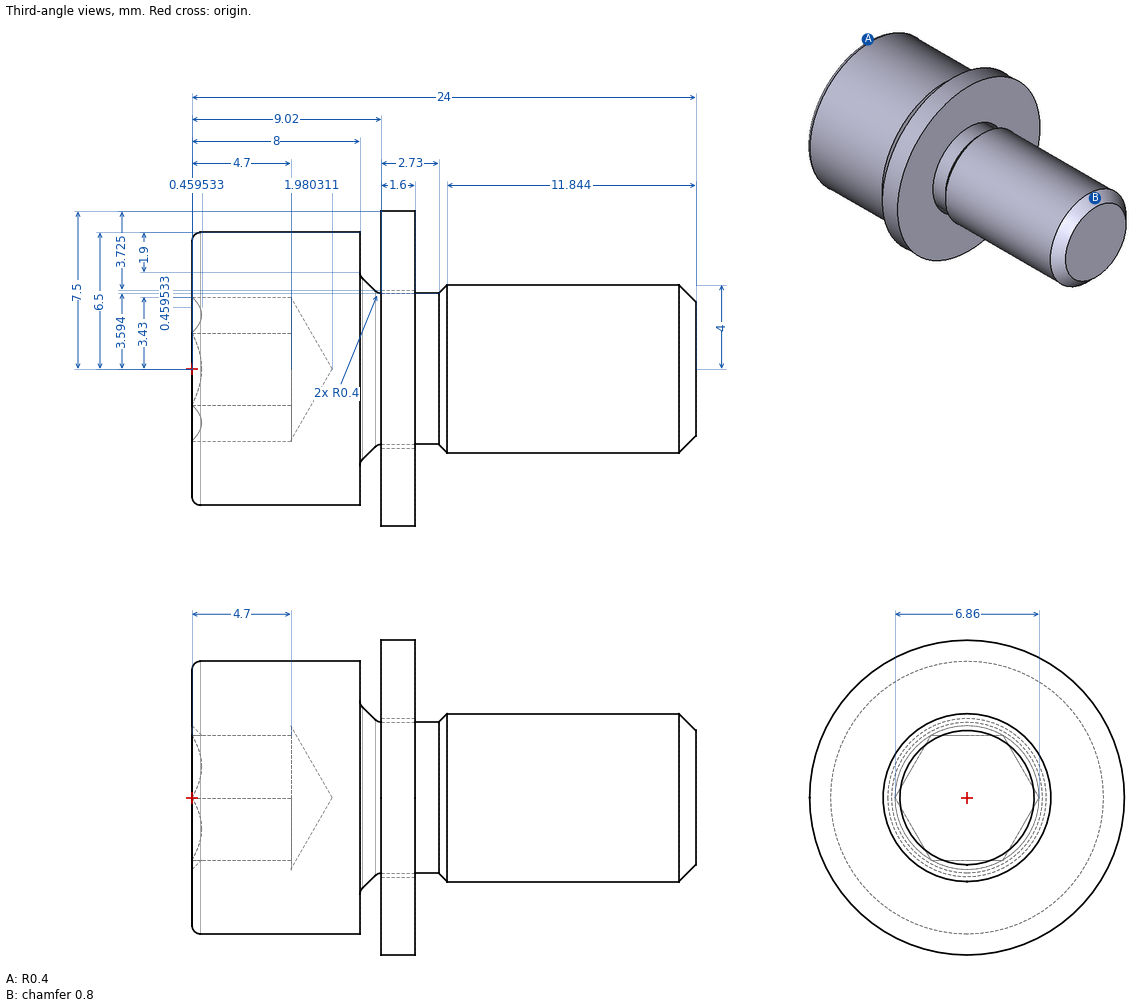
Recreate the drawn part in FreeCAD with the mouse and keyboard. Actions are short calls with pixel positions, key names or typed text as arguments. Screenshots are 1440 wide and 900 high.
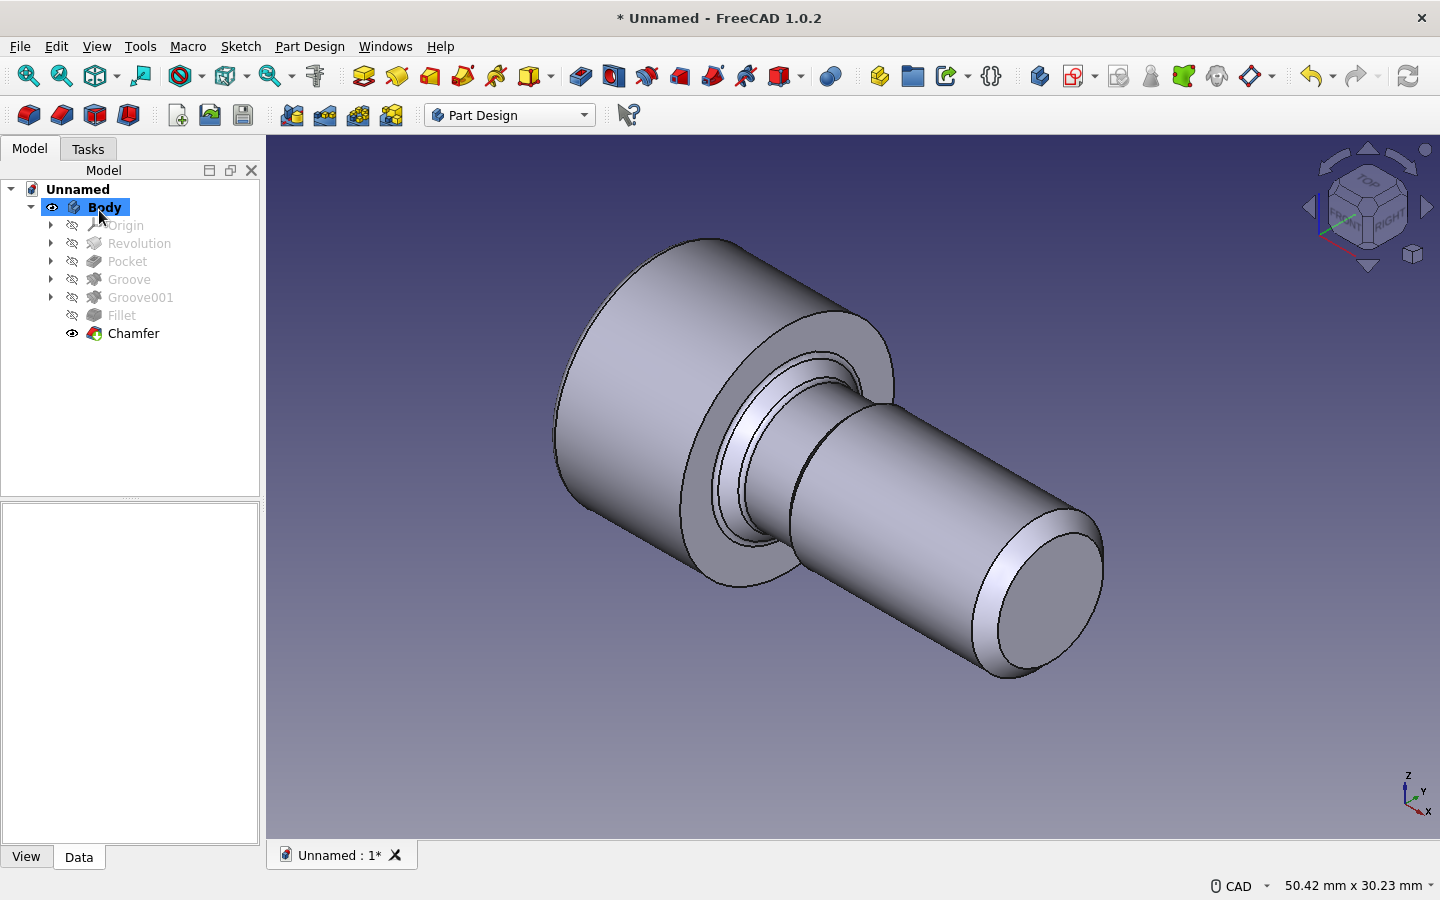
click(1040, 76)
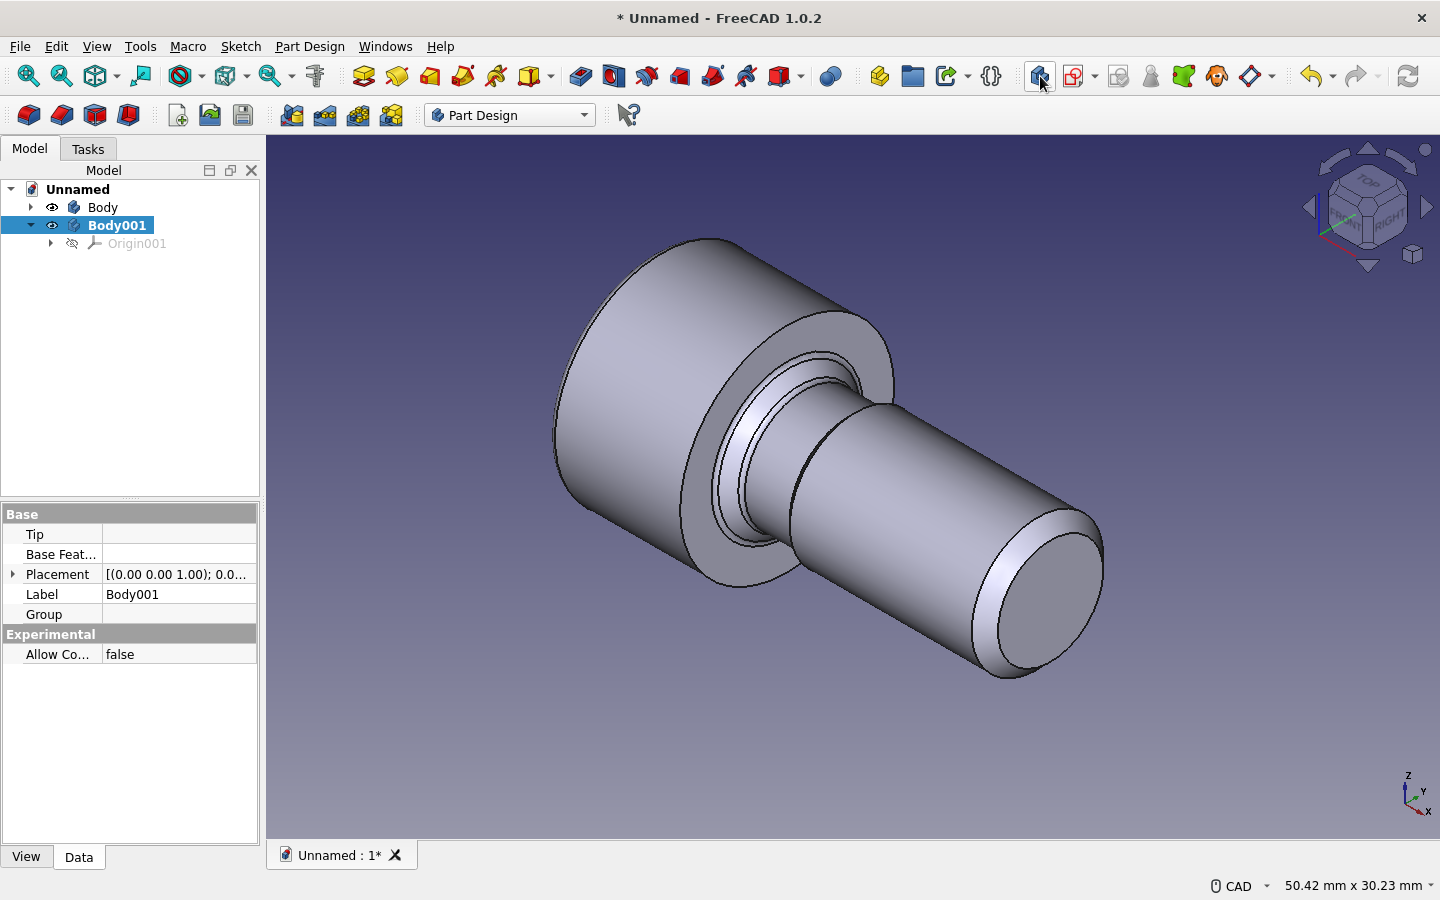
click(306, 799)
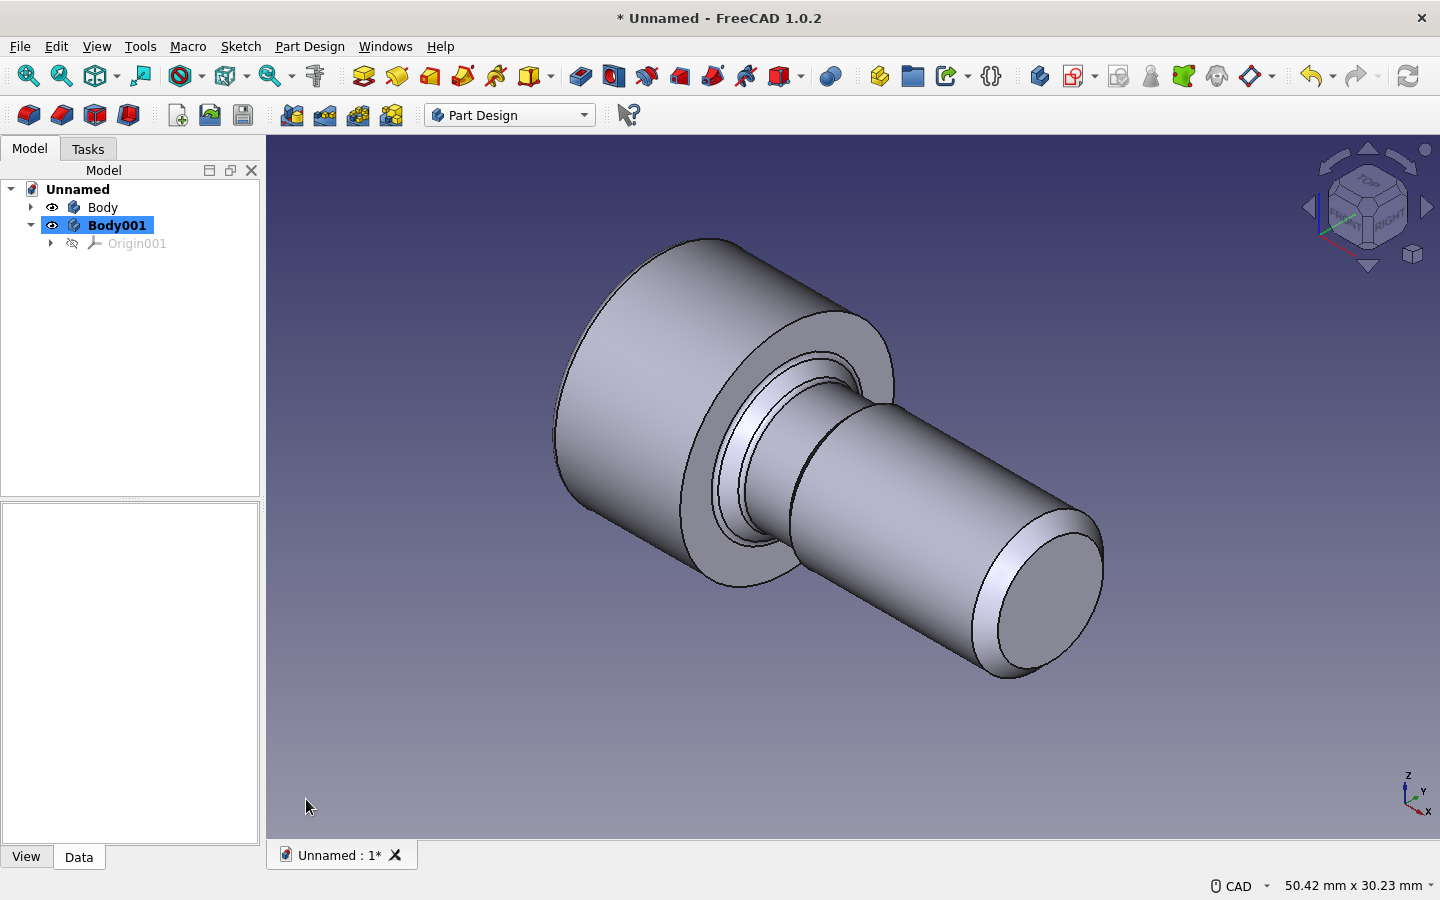
click(1072, 76)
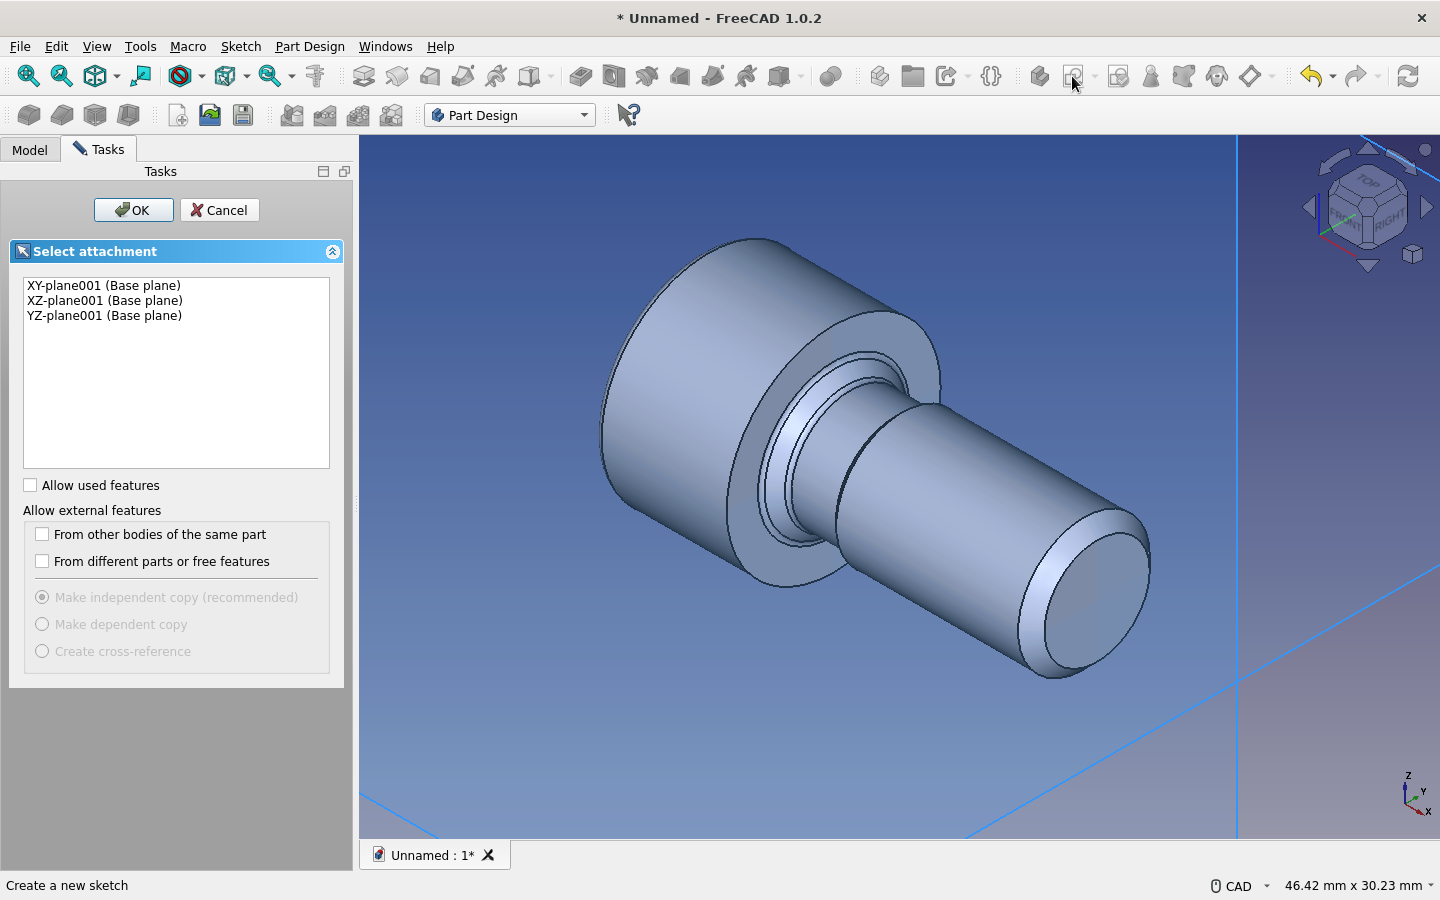
click(84, 286)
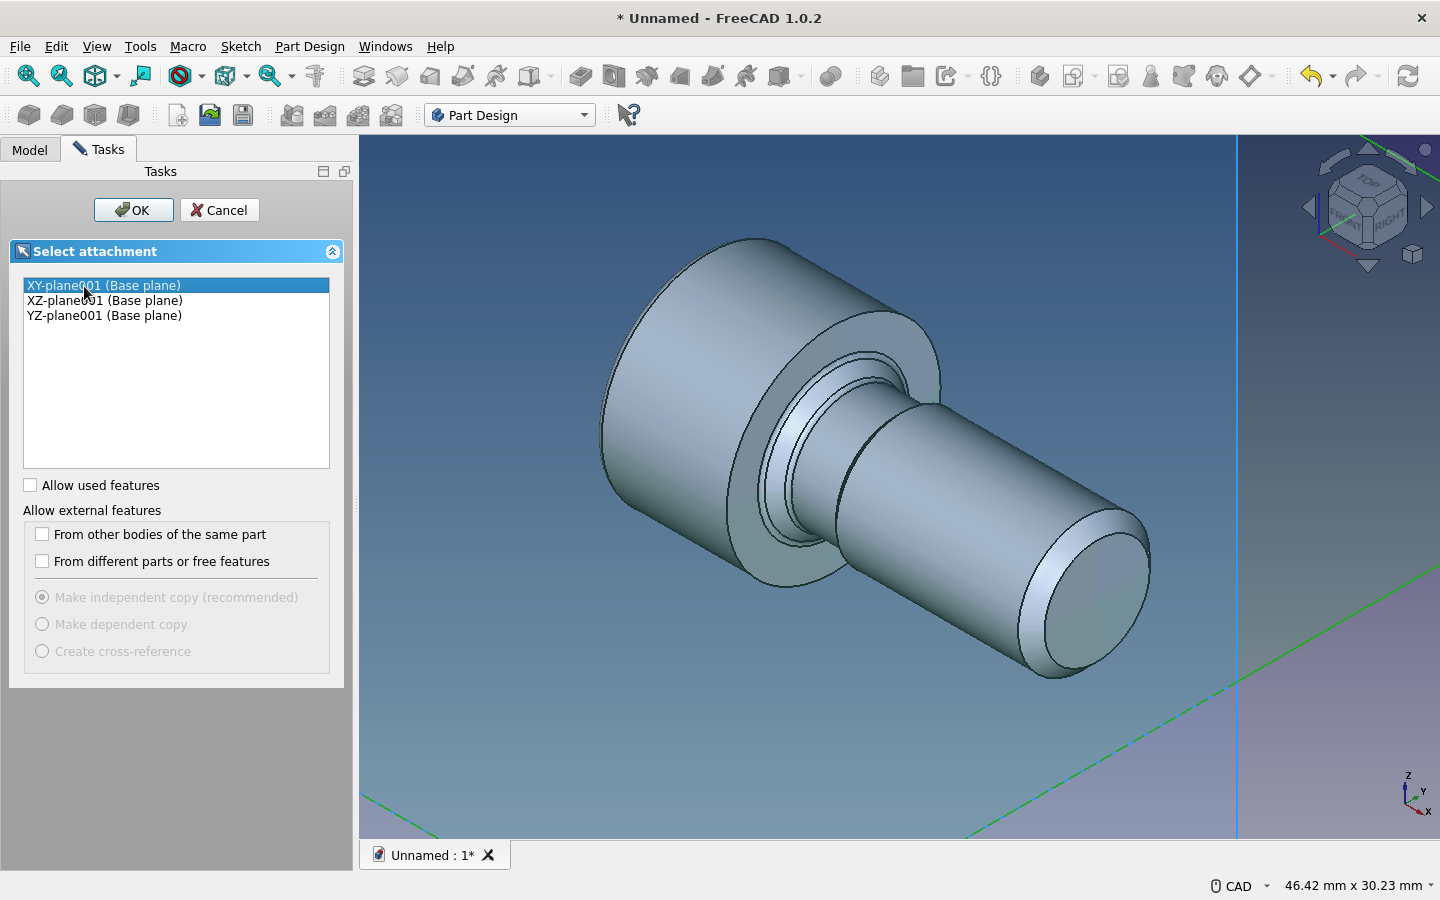
click(134, 210)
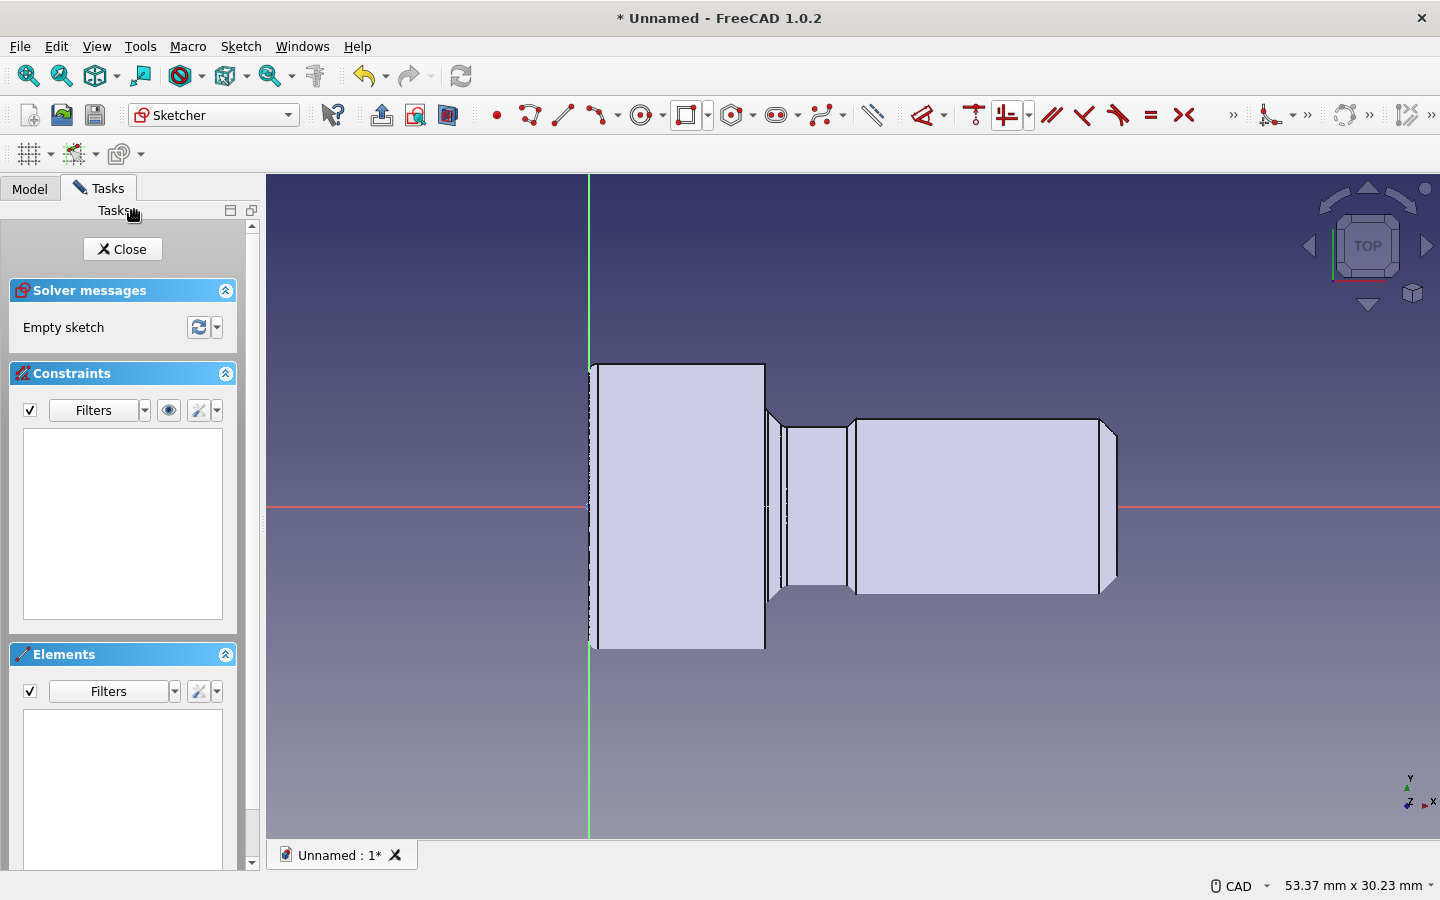
scroll(810, 351, up, 8)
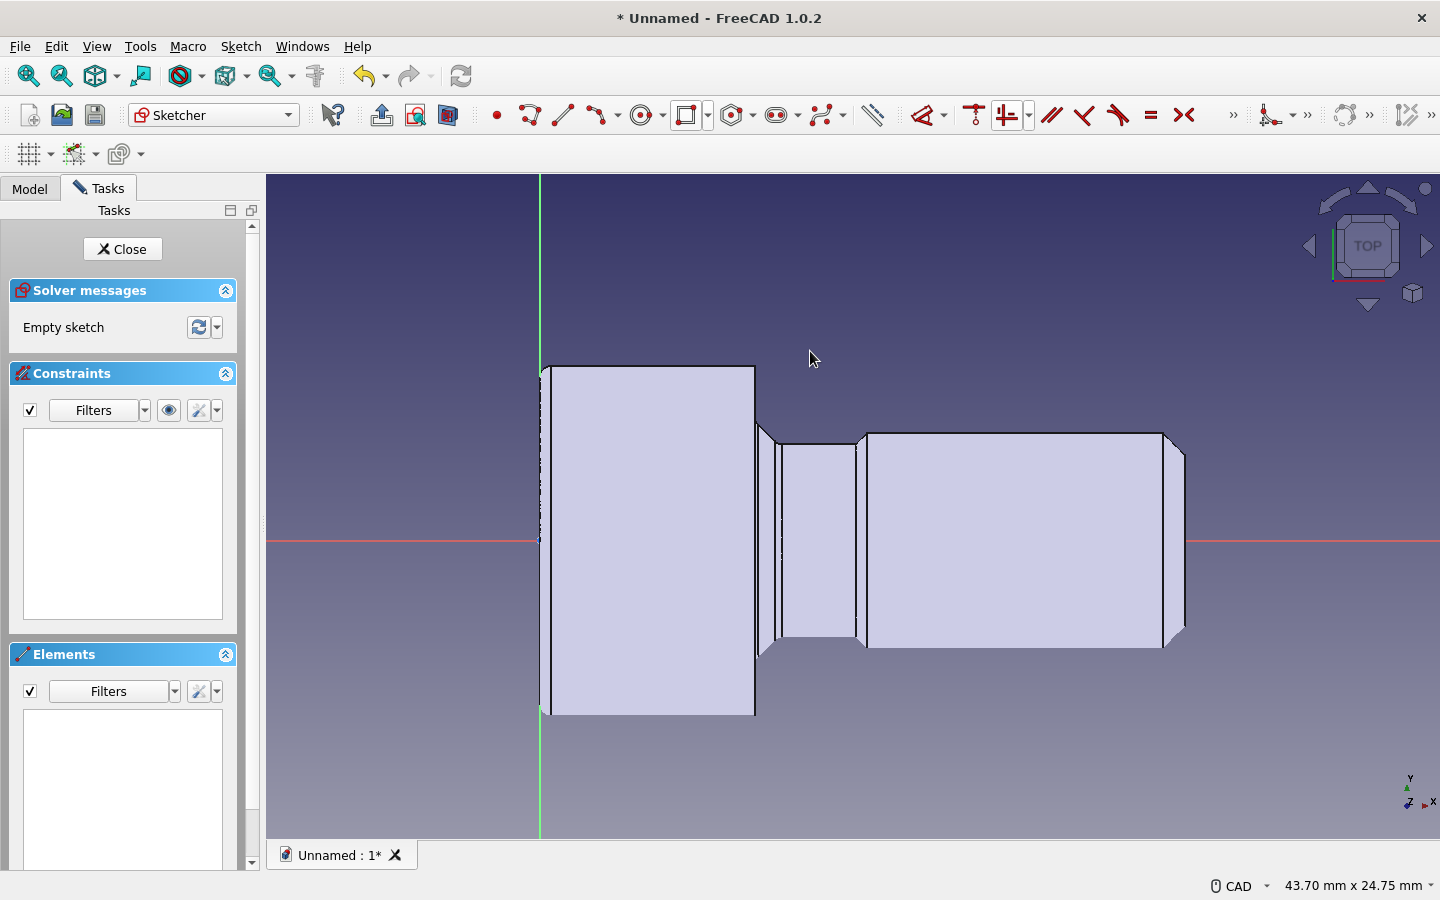
click(686, 116)